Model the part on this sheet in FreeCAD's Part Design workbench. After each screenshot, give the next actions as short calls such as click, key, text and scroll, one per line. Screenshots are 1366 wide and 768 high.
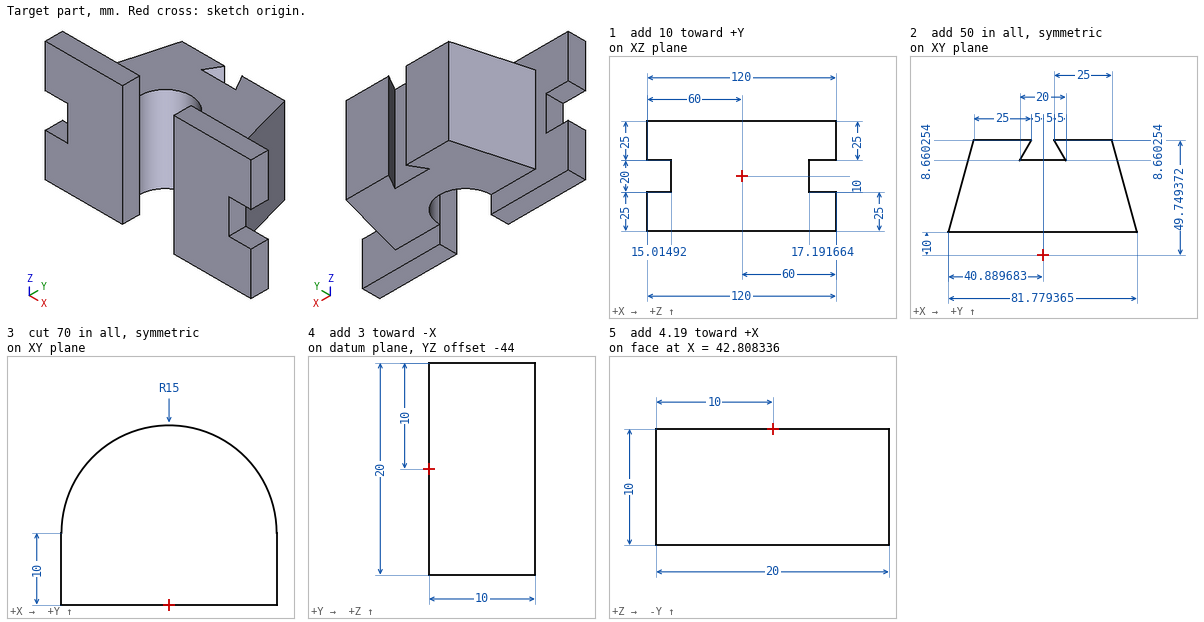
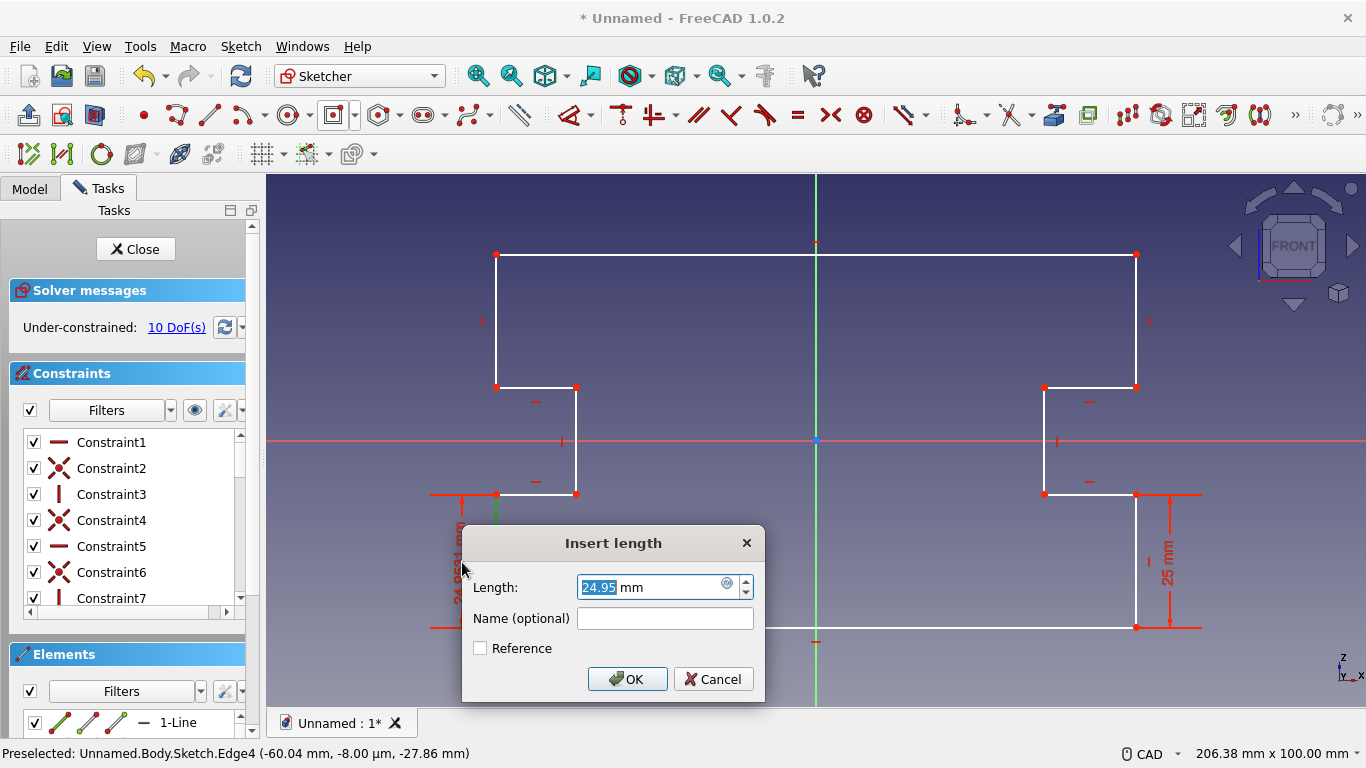
text(25)
key(Return)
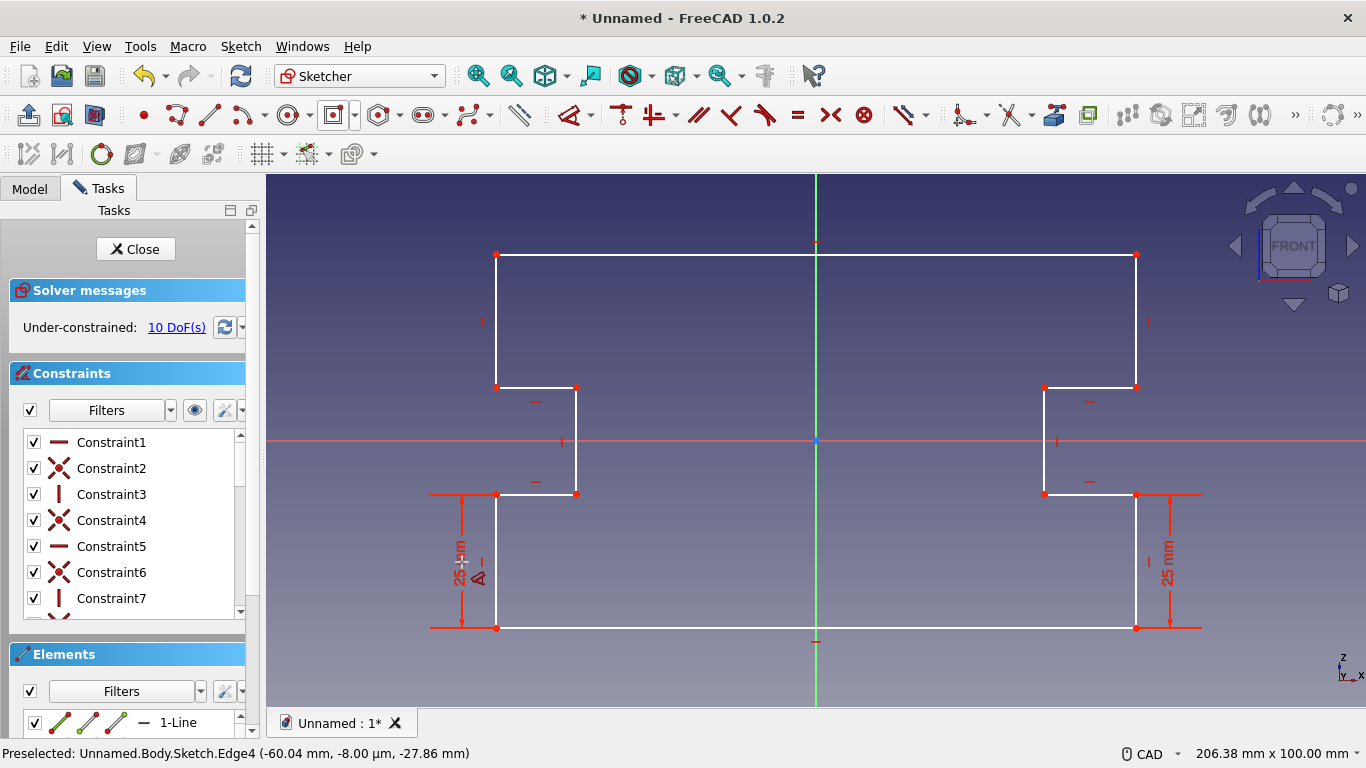
click(576, 463)
click(542, 417)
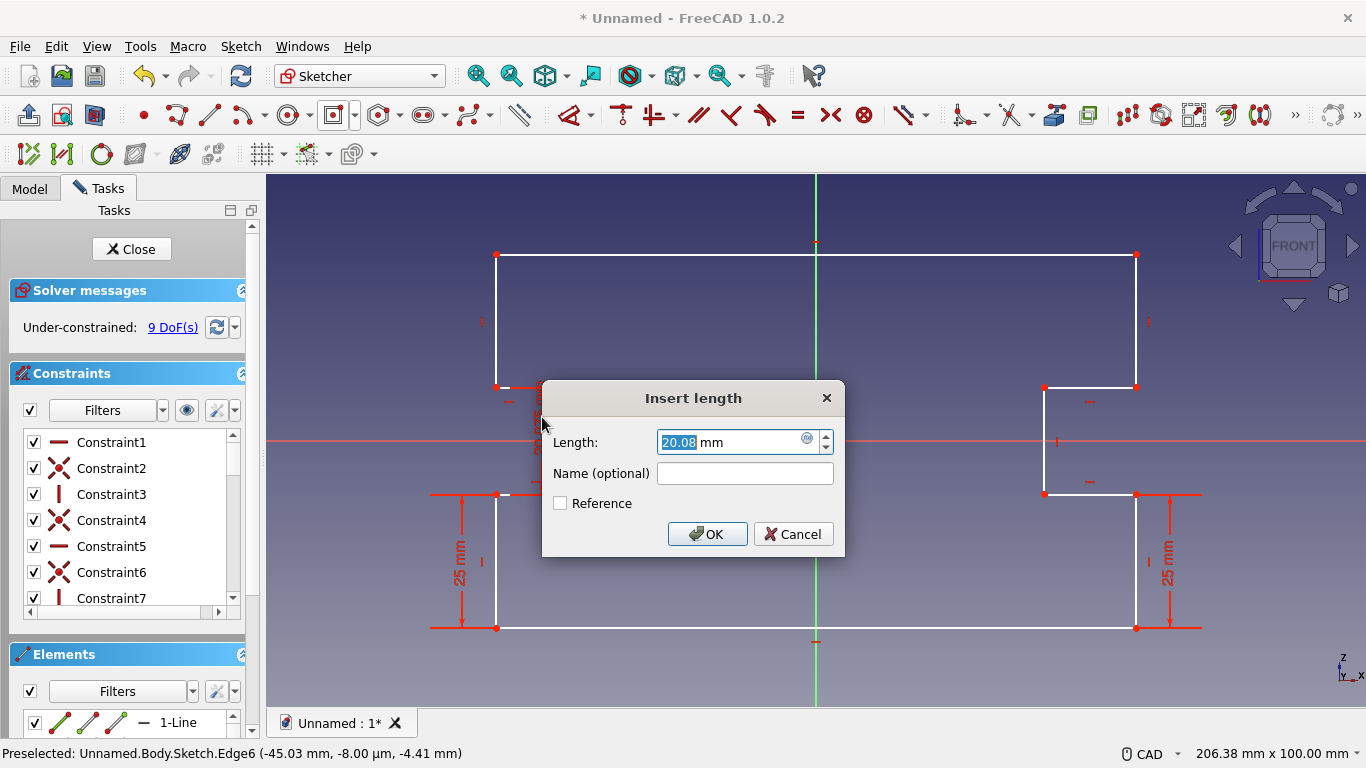
text(20)
key(Return)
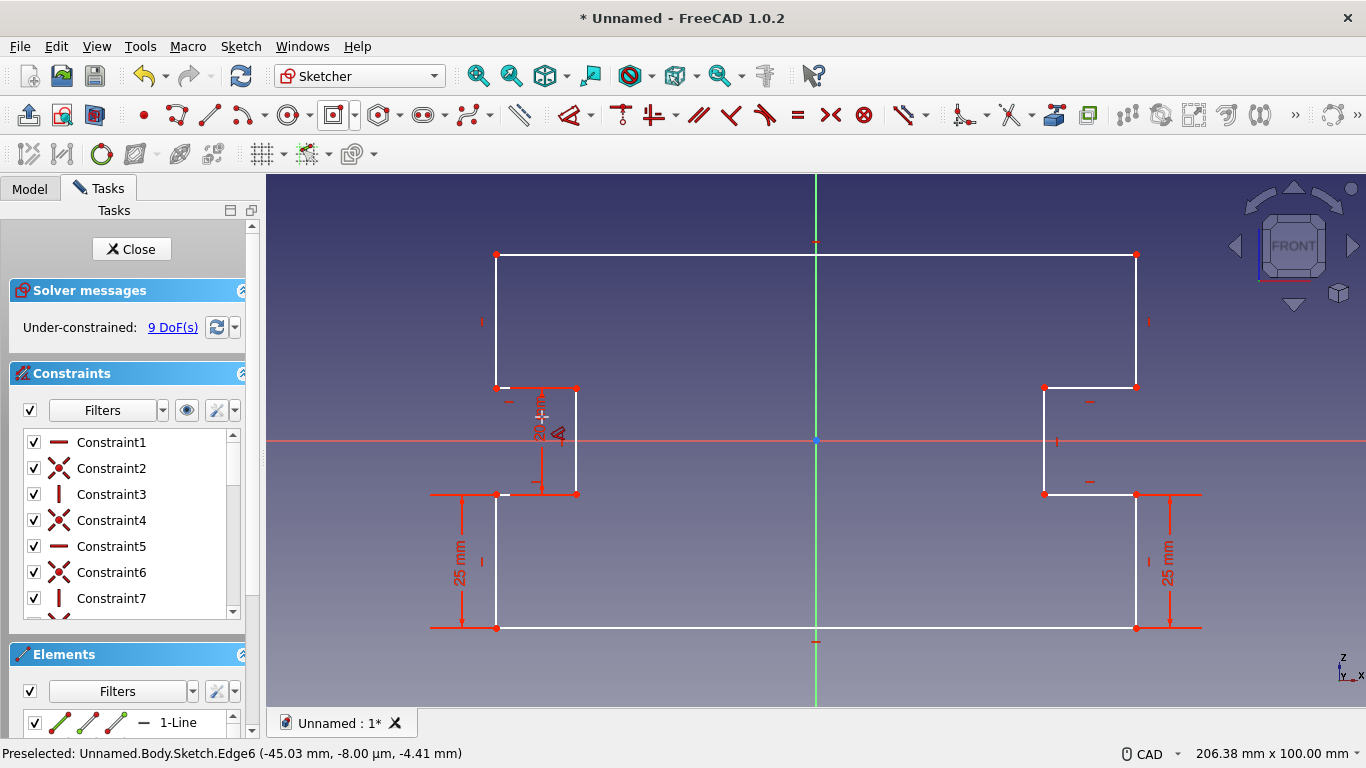
click(496, 348)
click(462, 322)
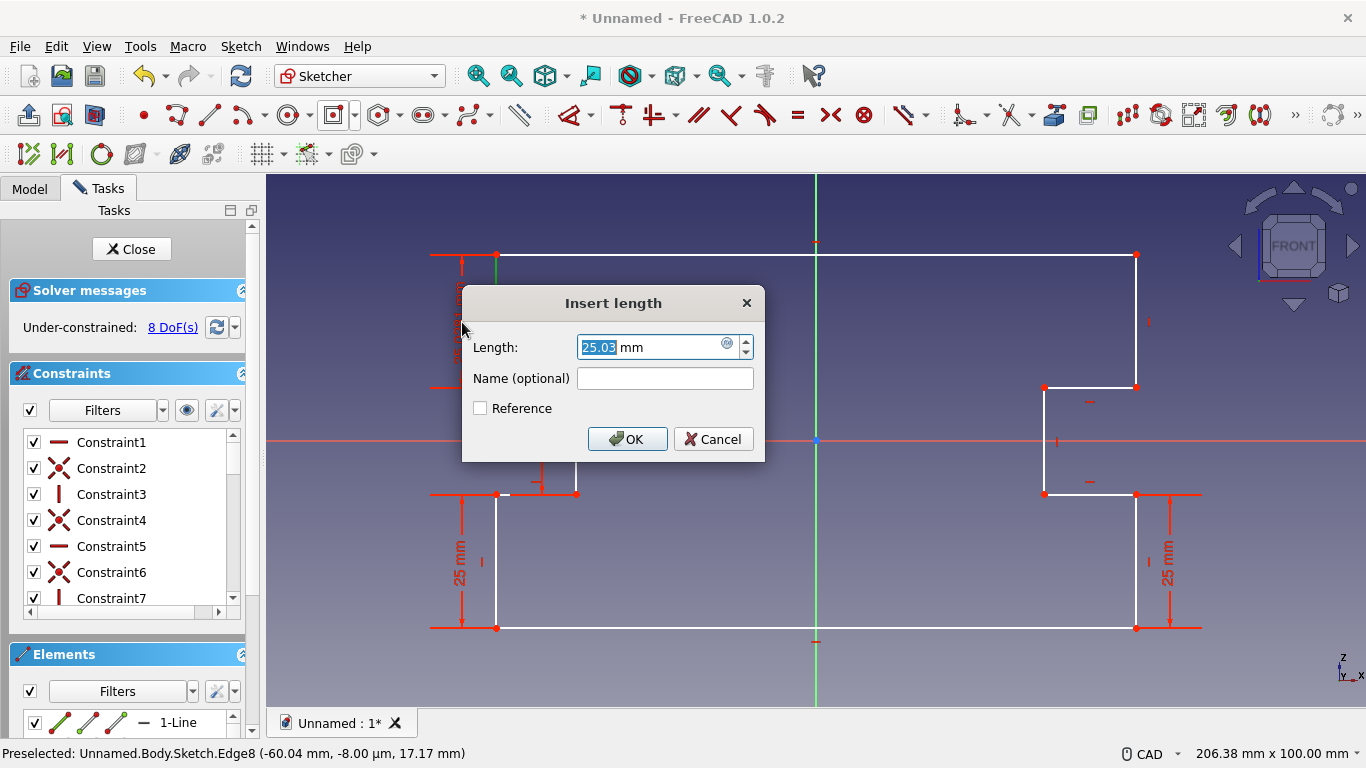
text(25)
key(Return)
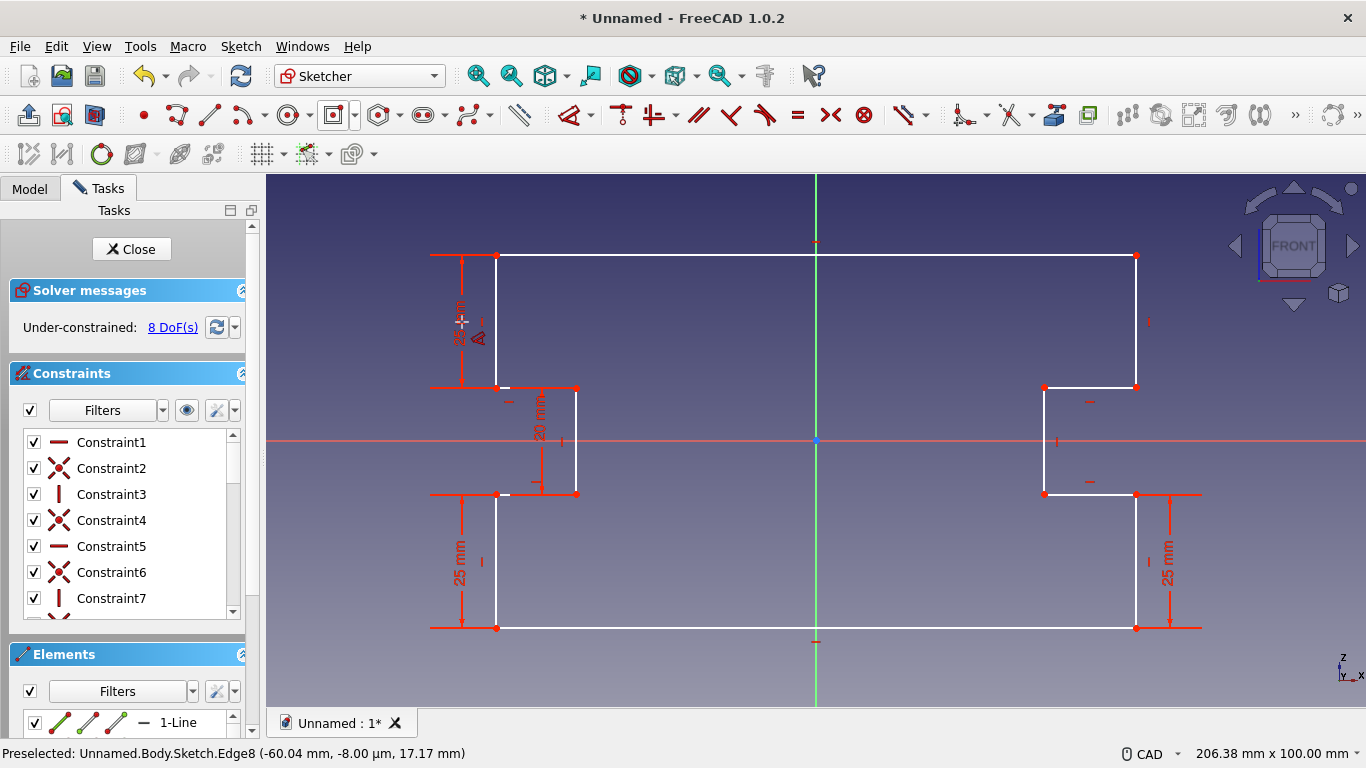
click(1136, 295)
click(1170, 322)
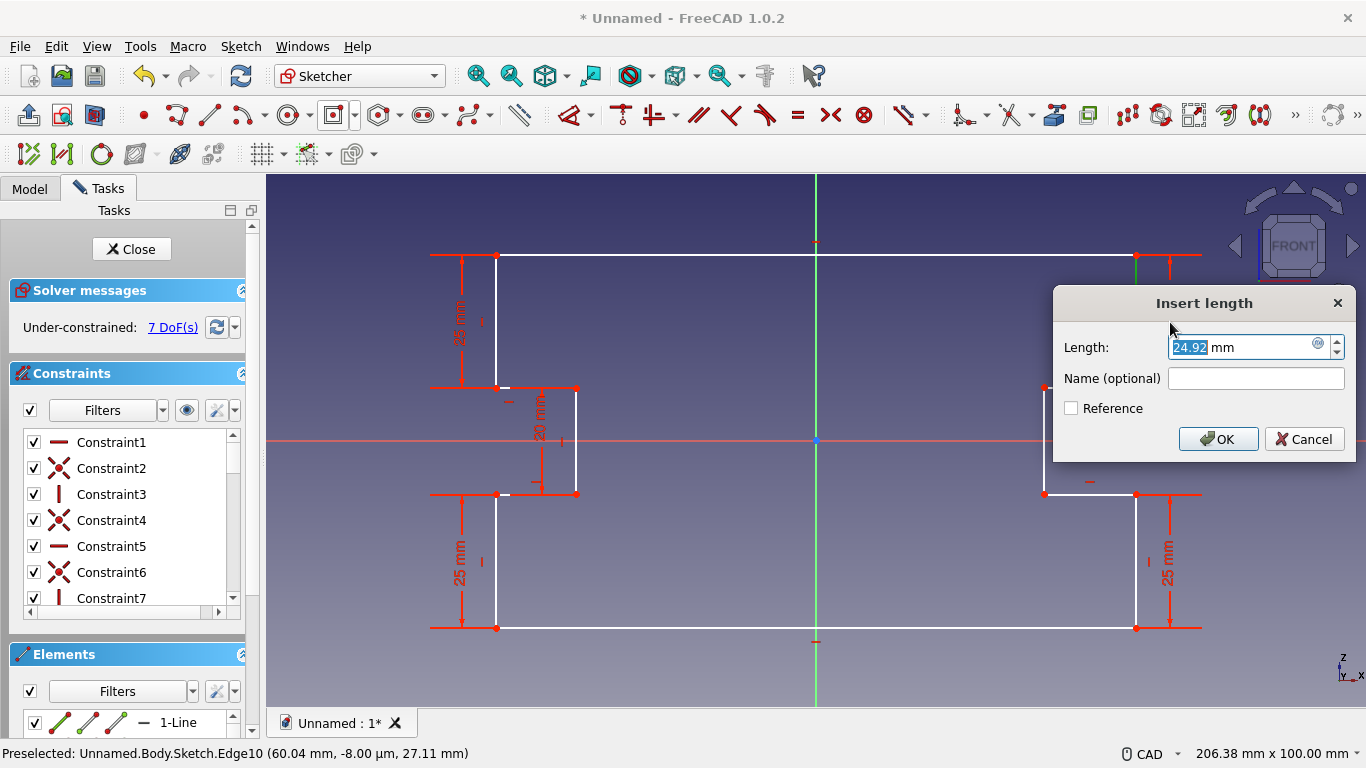
text(25)
key(Return)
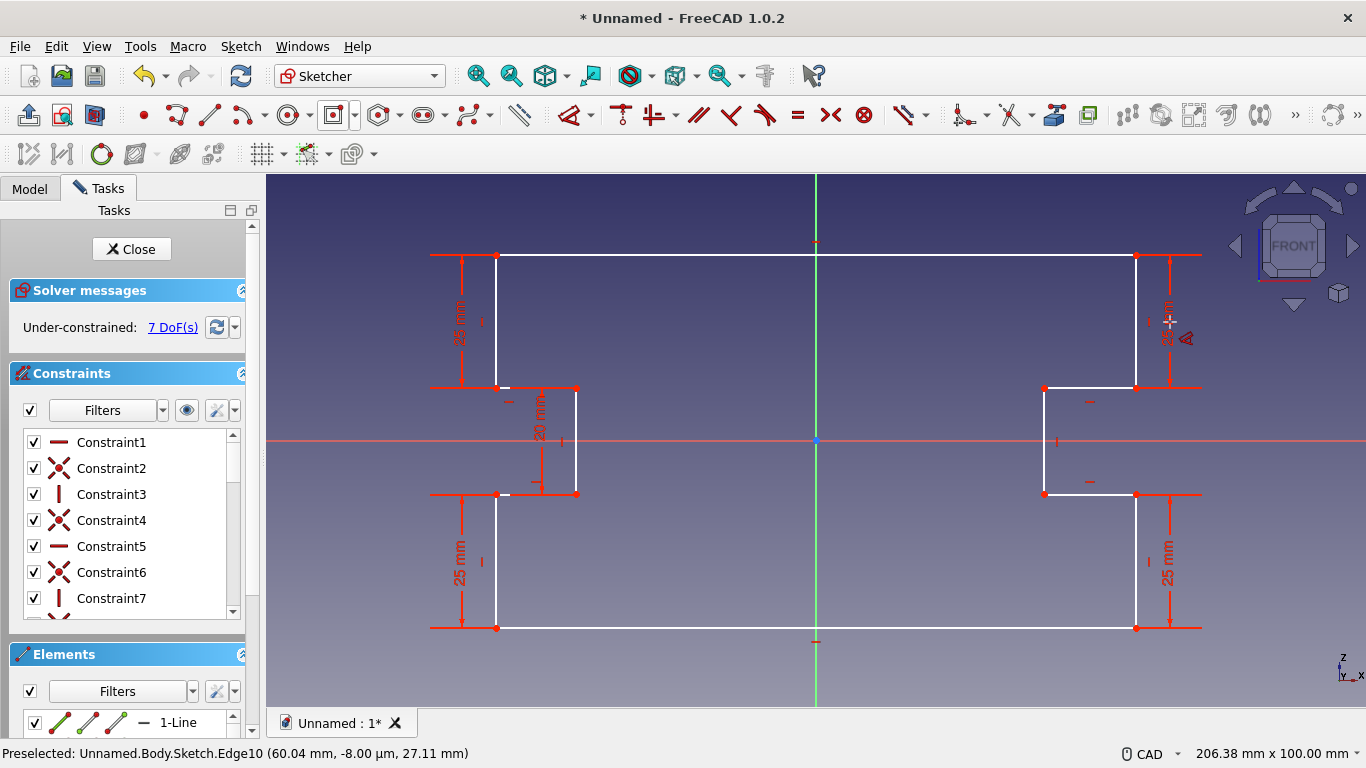
click(944, 628)
click(669, 662)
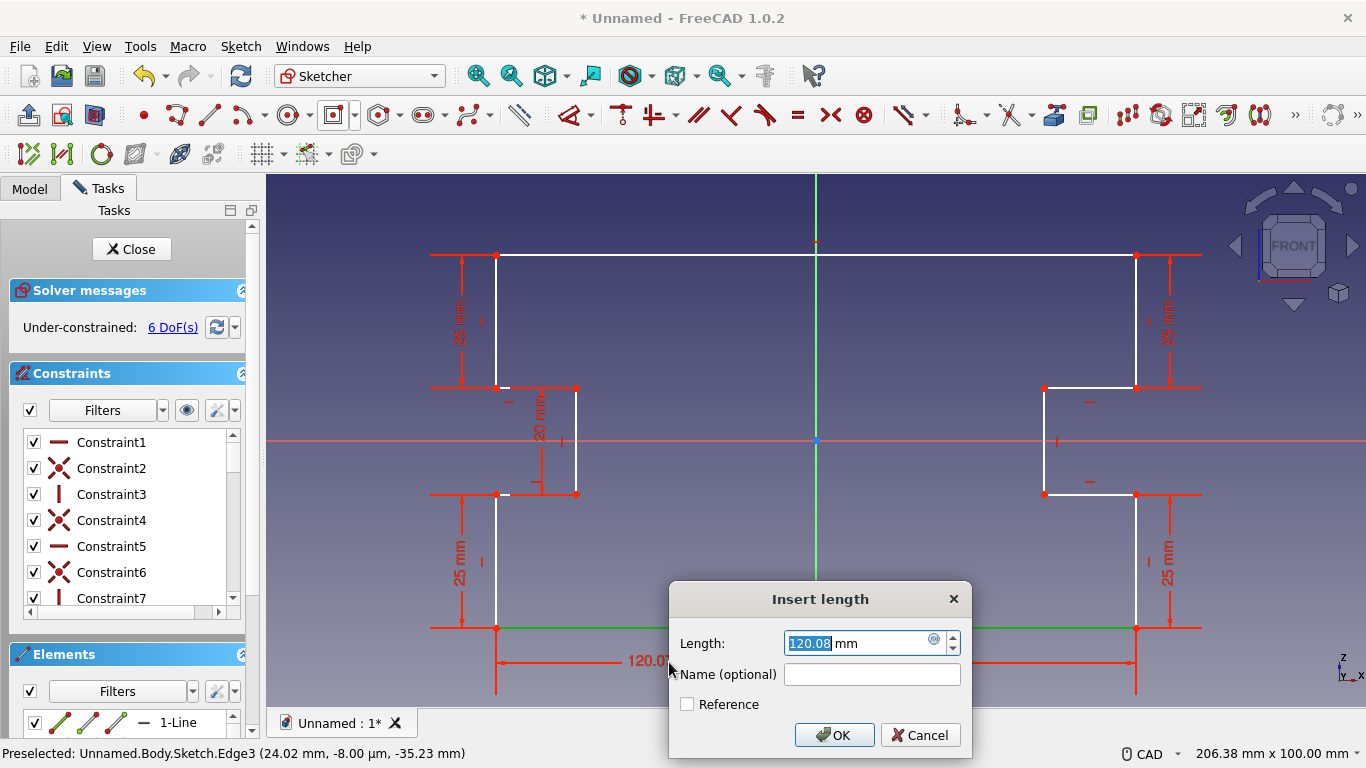
text(120)
key(Return)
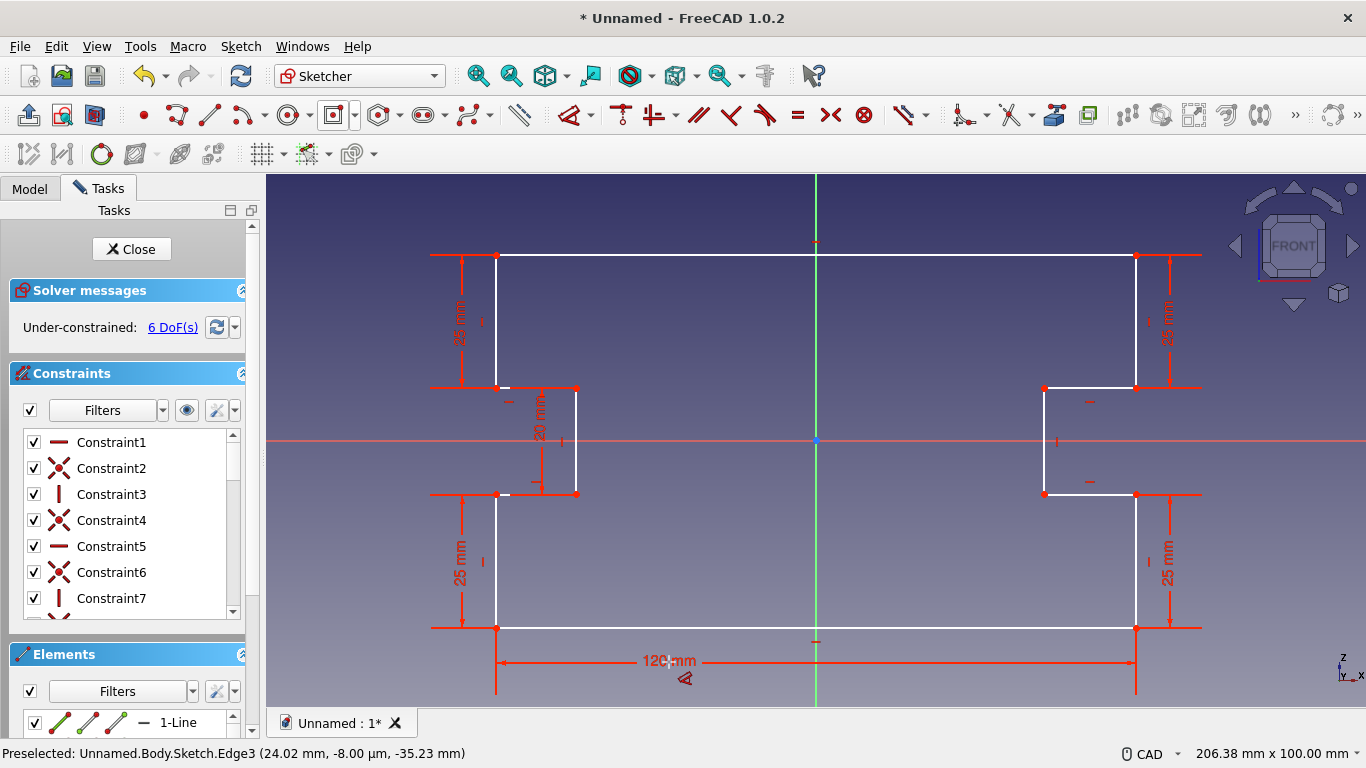
click(688, 255)
click(669, 221)